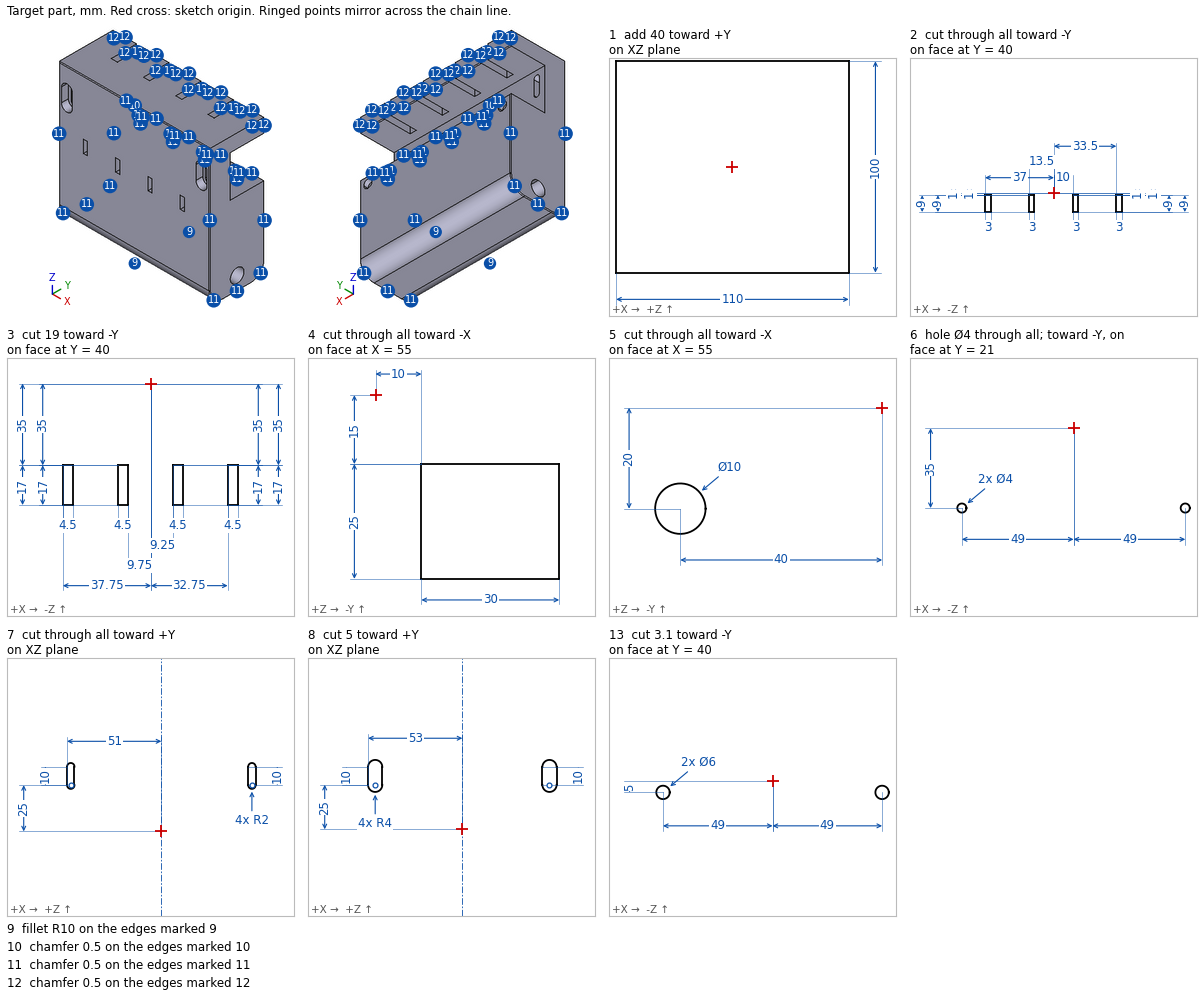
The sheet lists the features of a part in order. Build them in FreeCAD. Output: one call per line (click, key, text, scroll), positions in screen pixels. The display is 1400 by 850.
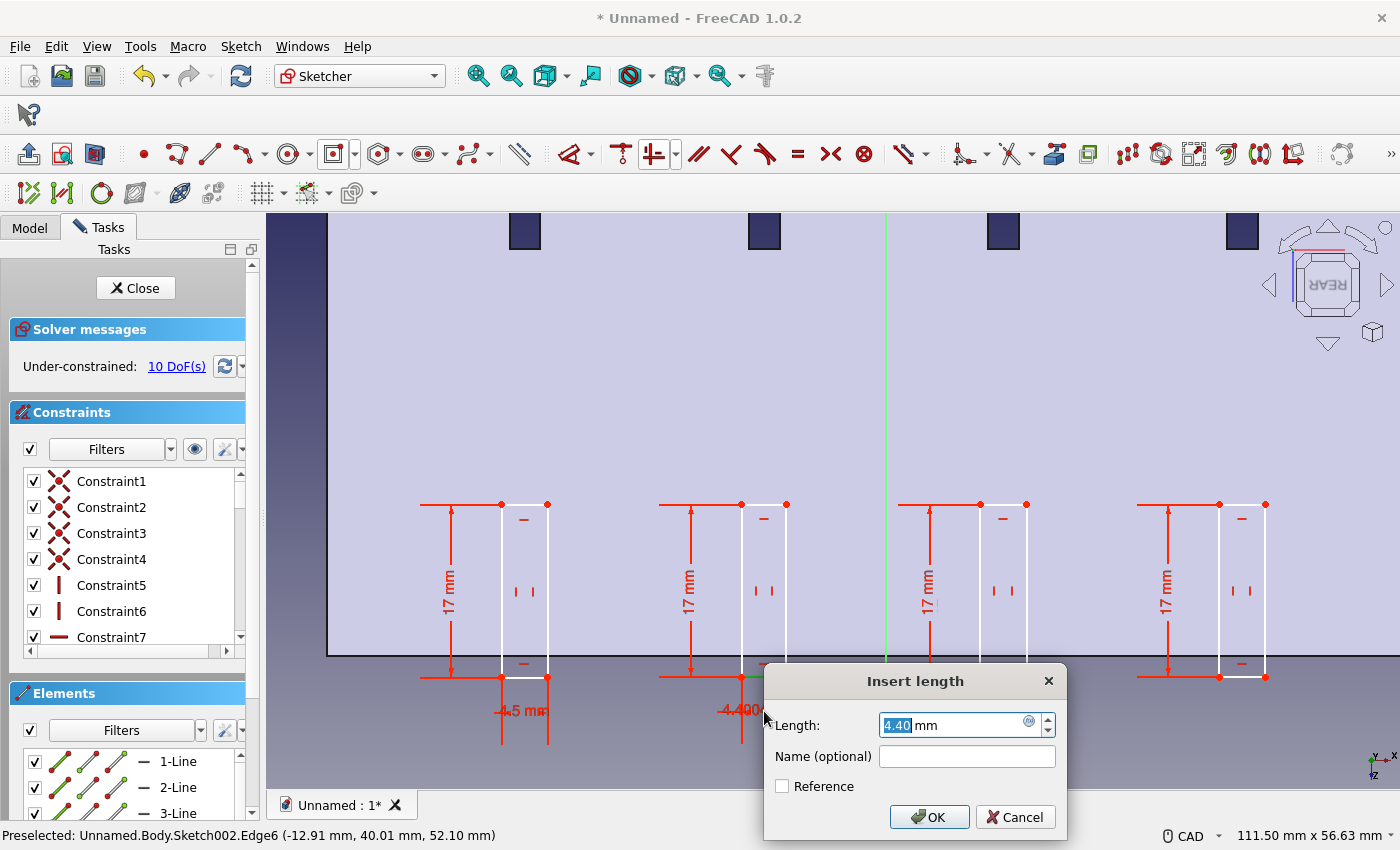
text(4.5)
key(Return)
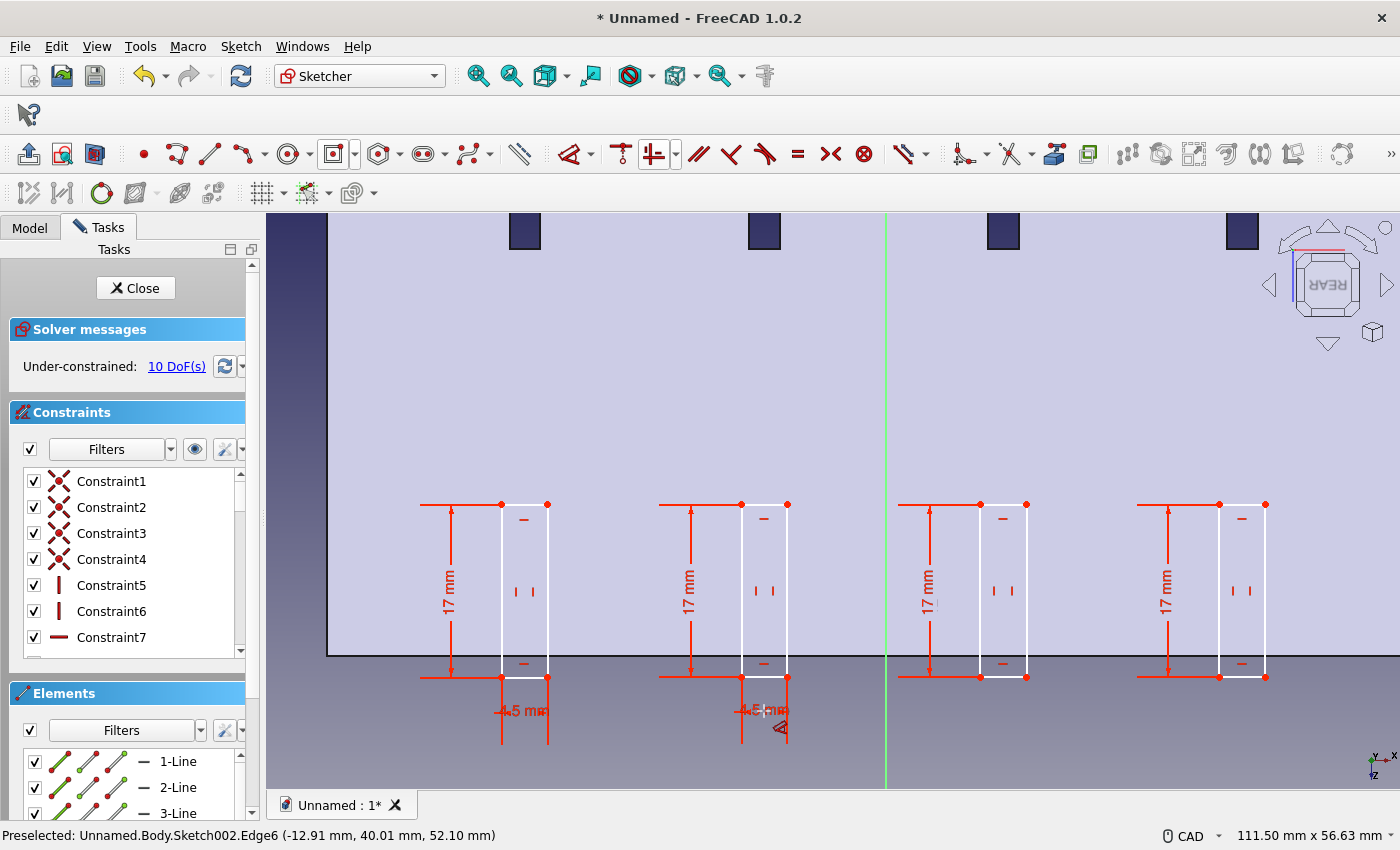
click(994, 677)
click(1003, 711)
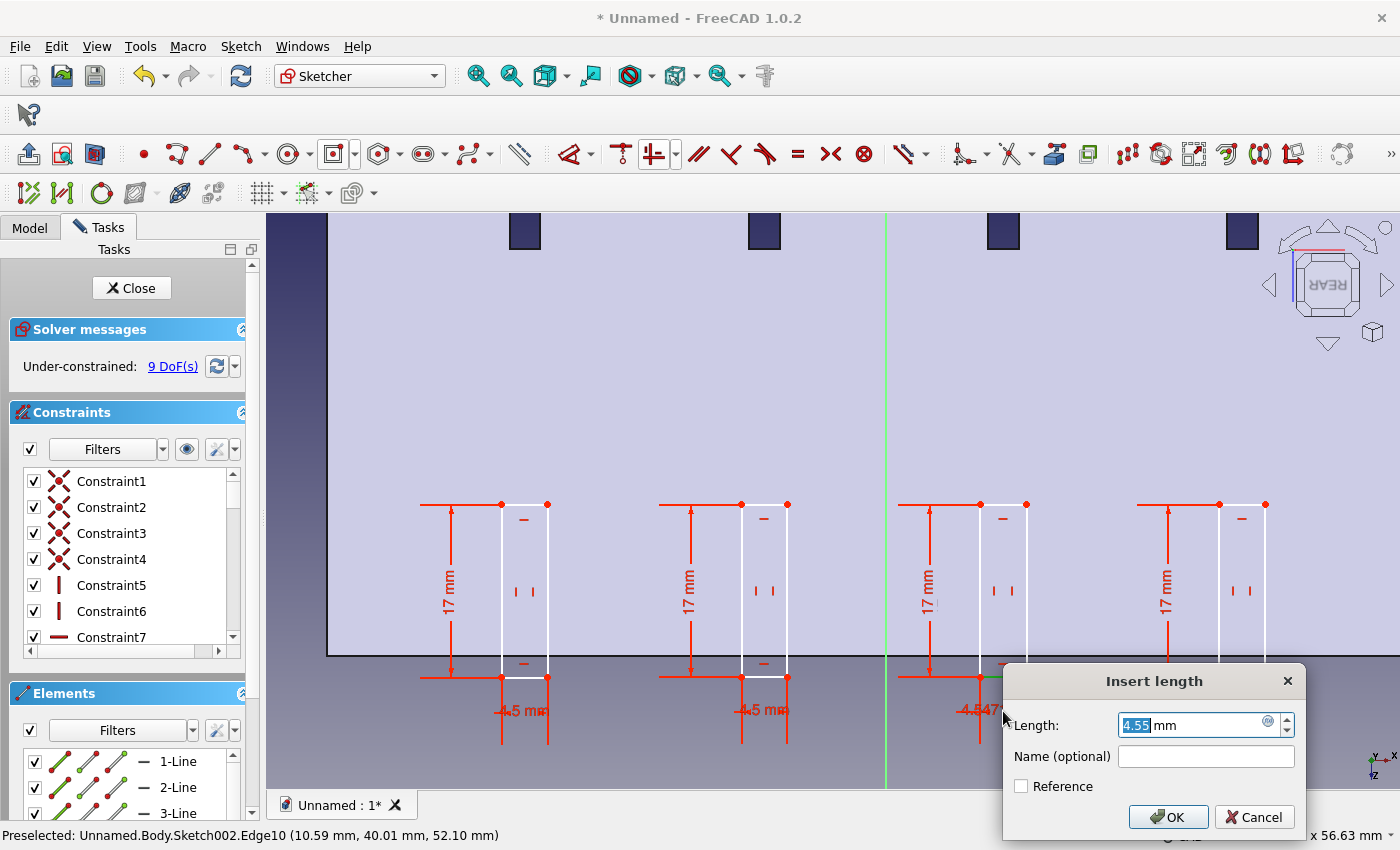
text(4.5)
key(Return)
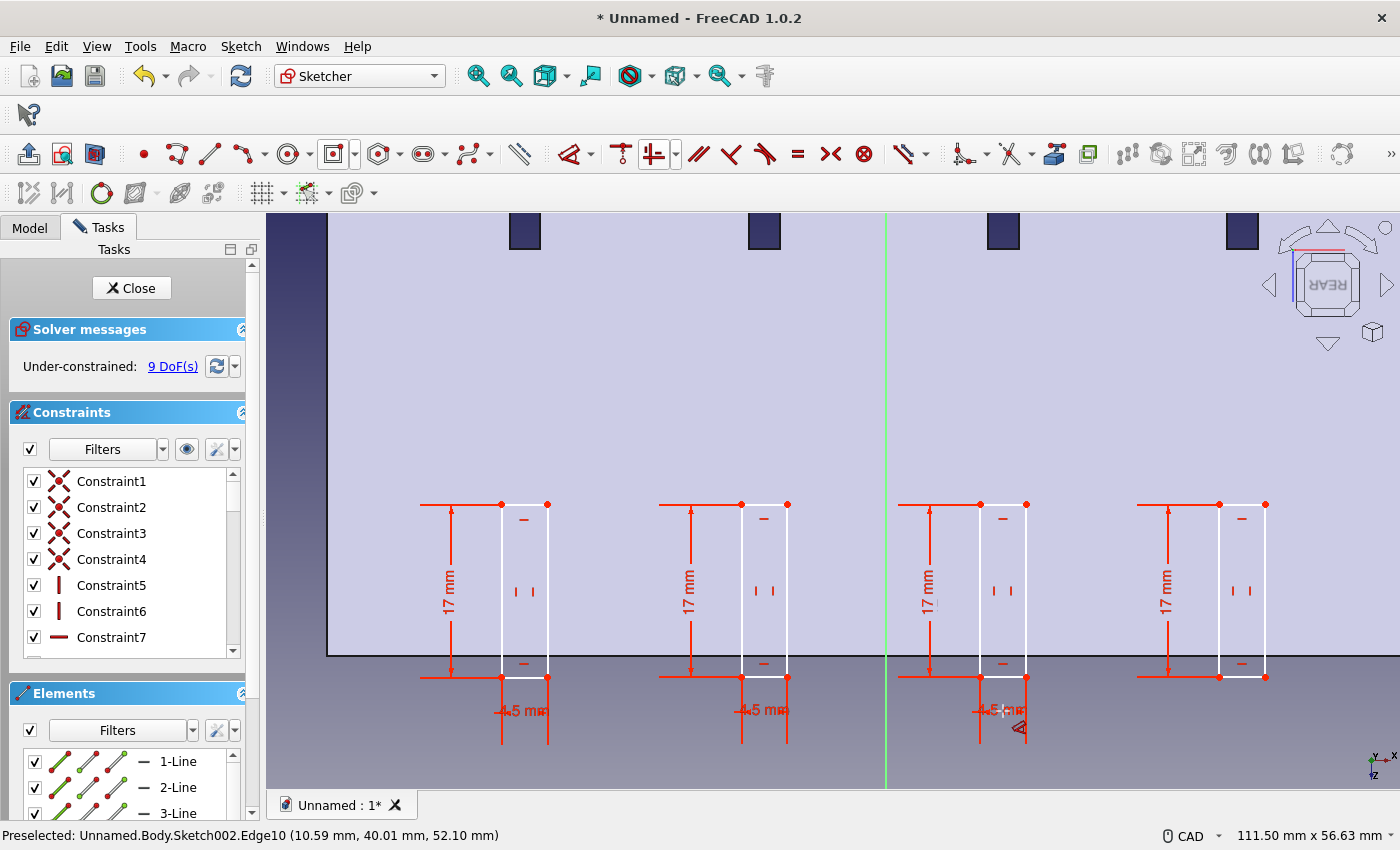
click(1233, 677)
click(1227, 711)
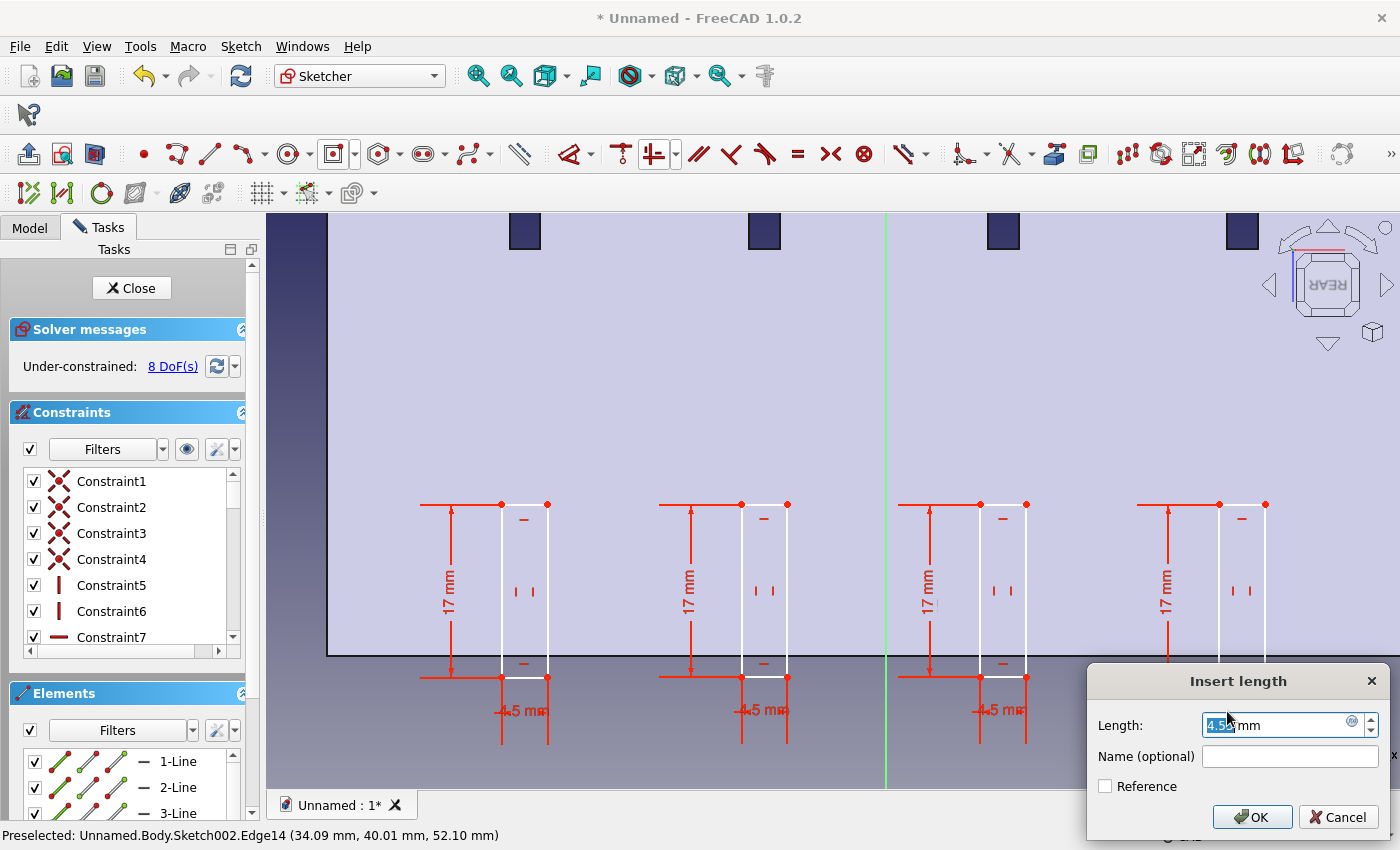
text(4.5)
key(Return)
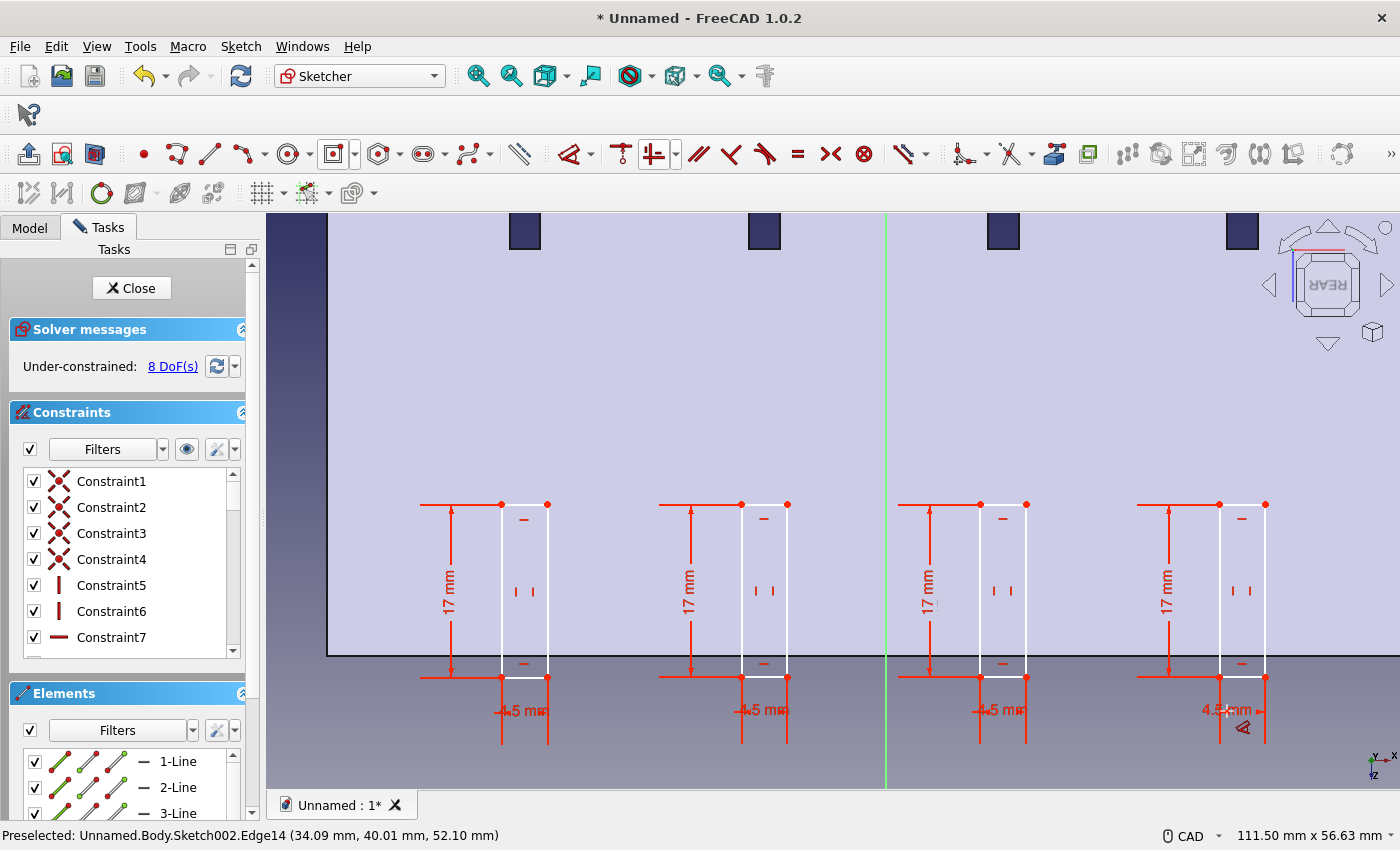
click(502, 505)
click(468, 373)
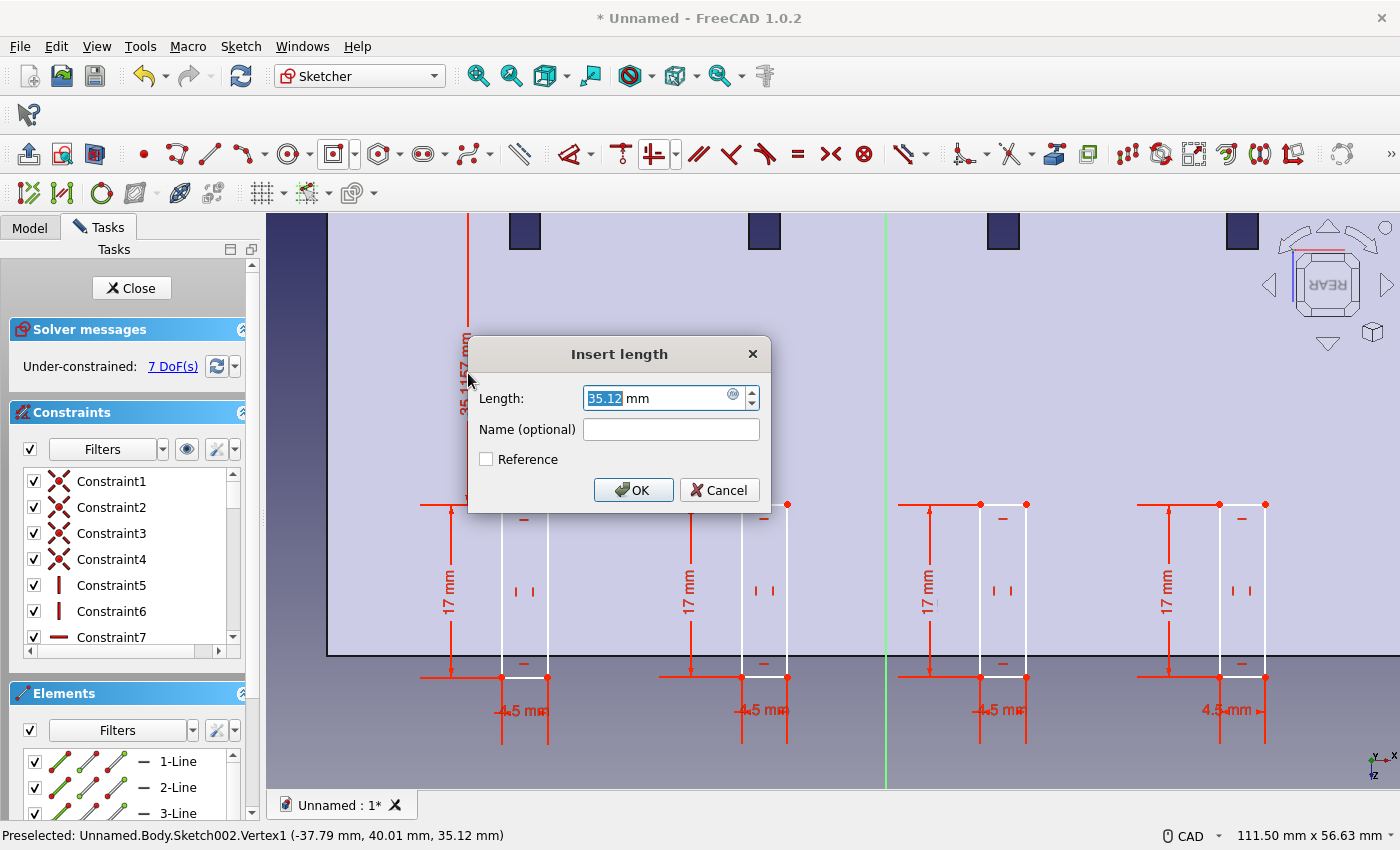
text(35)
key(Return)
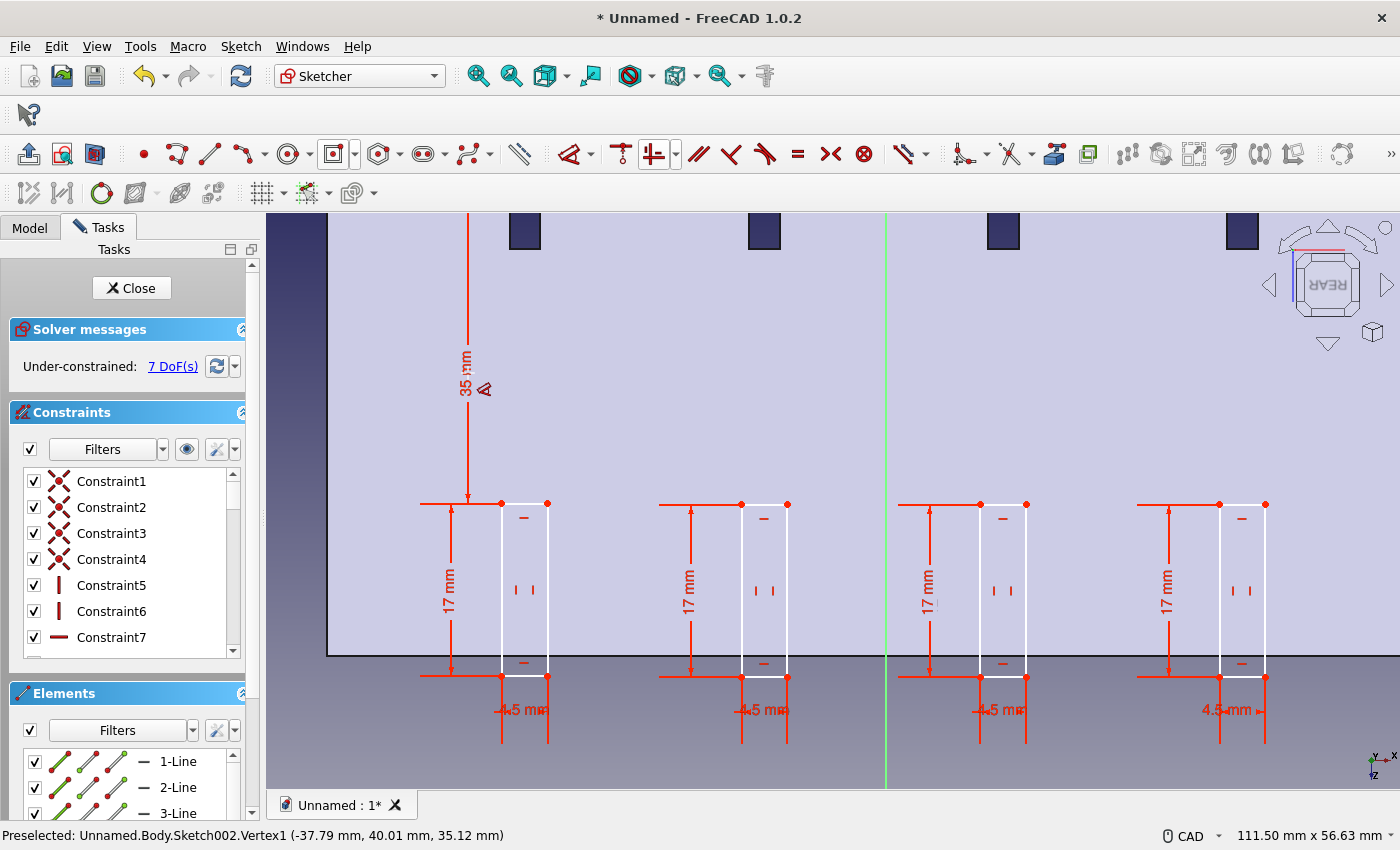
click(742, 505)
click(708, 373)